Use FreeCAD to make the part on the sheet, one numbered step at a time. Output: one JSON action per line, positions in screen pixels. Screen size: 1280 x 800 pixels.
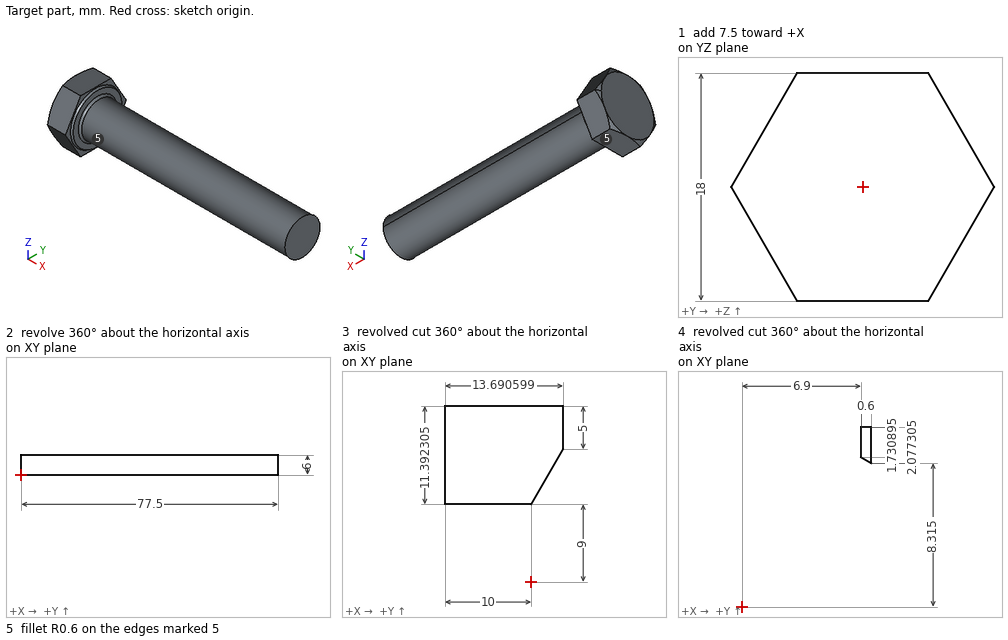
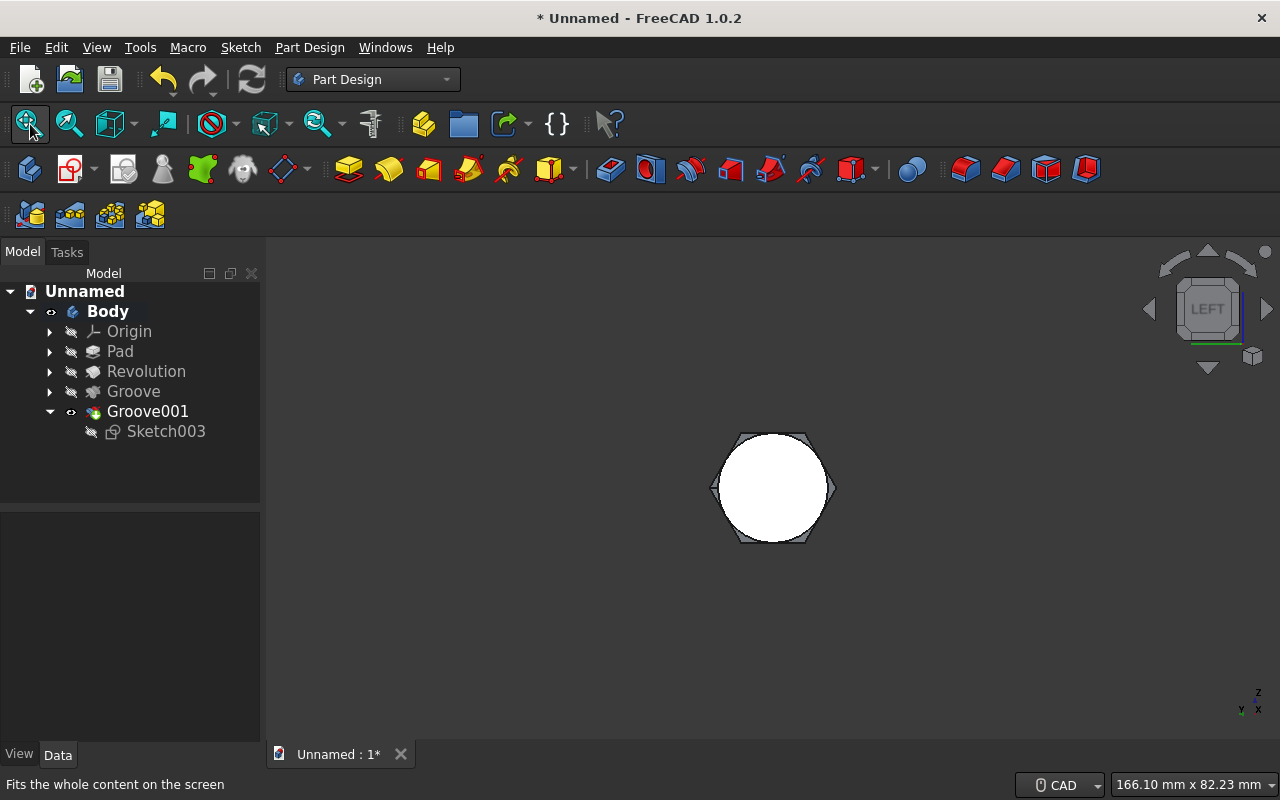
{"action": "left_click", "coordinate": [30, 124]}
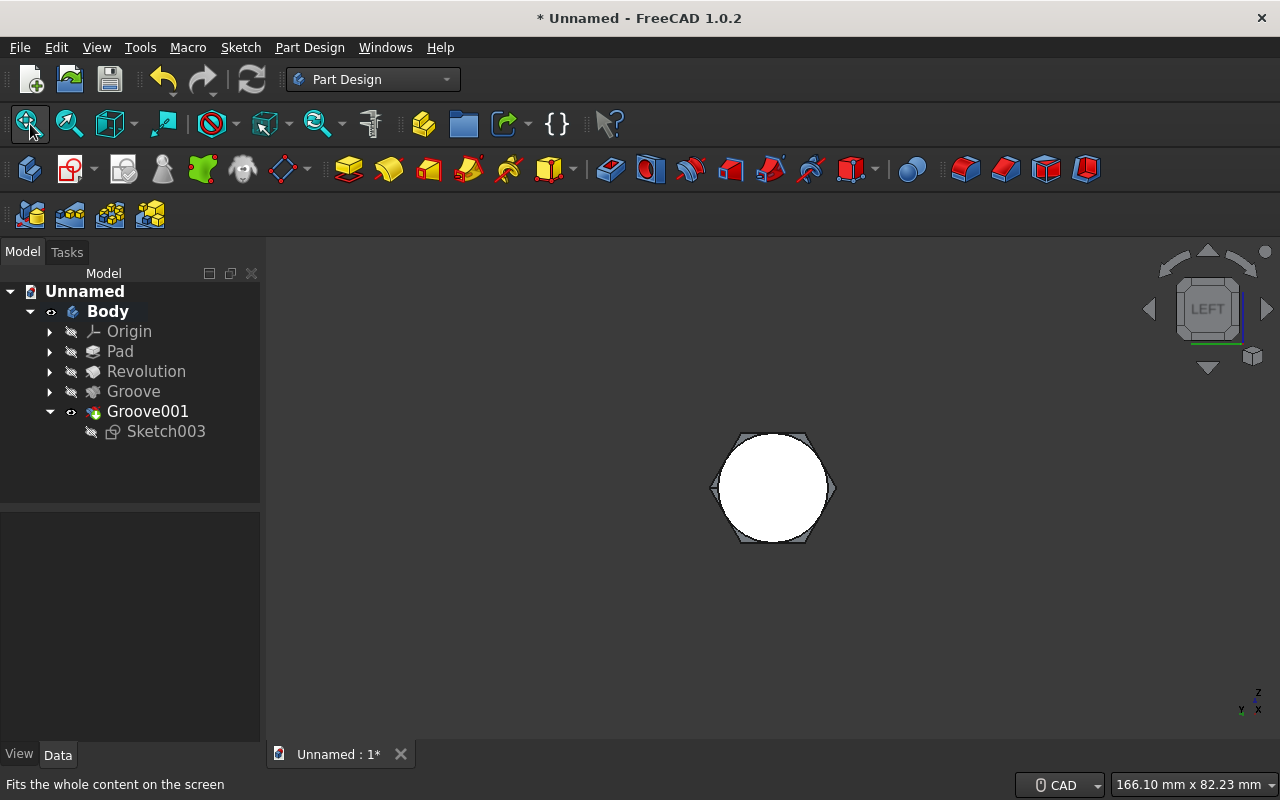
{"action": "key", "text": "v 3"}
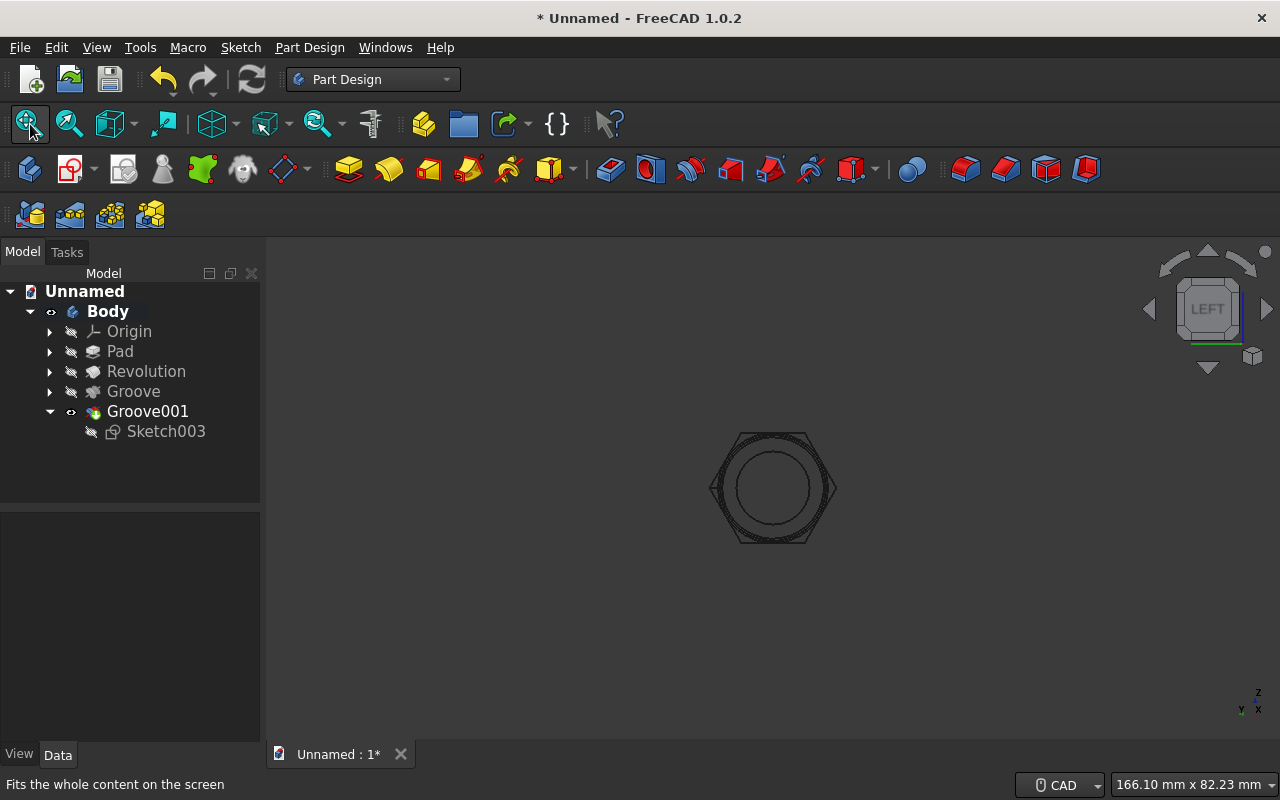
{"action": "key", "text": "0"}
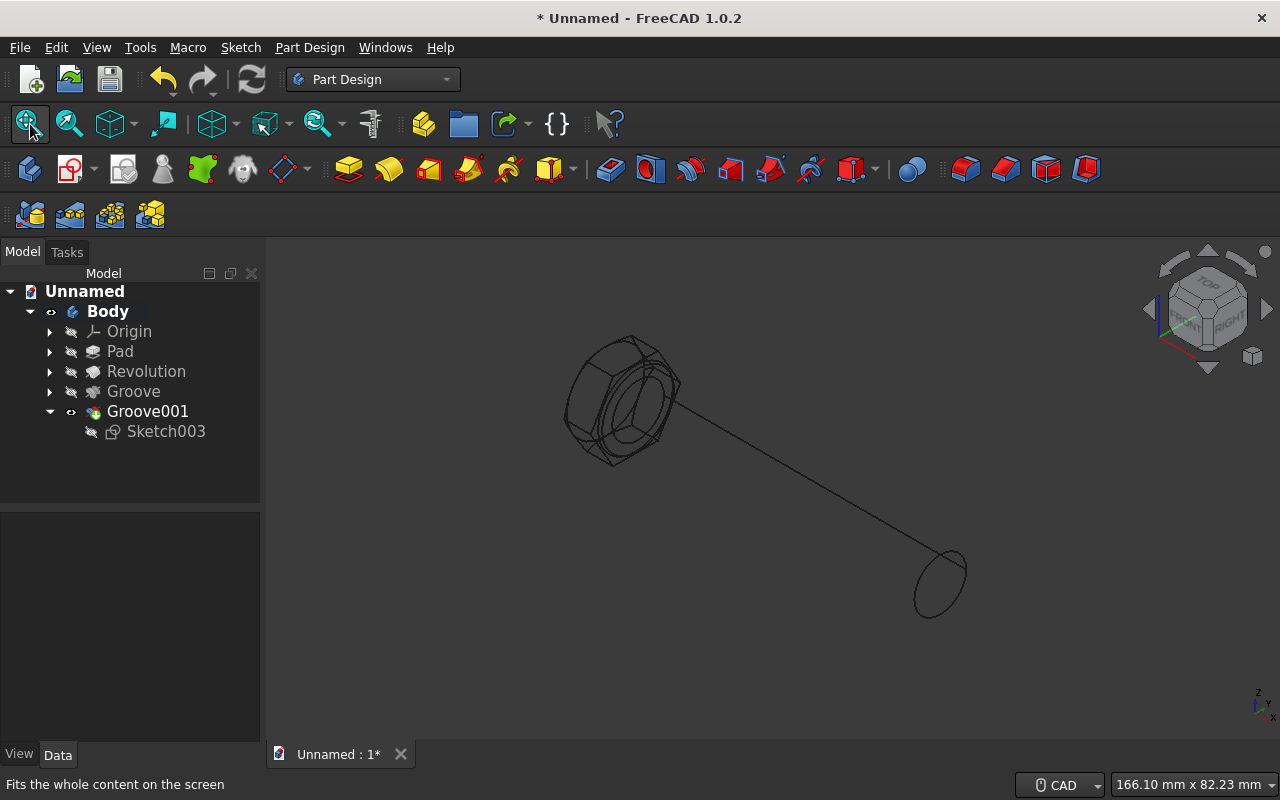
{"action": "left_click", "coordinate": [612, 424]}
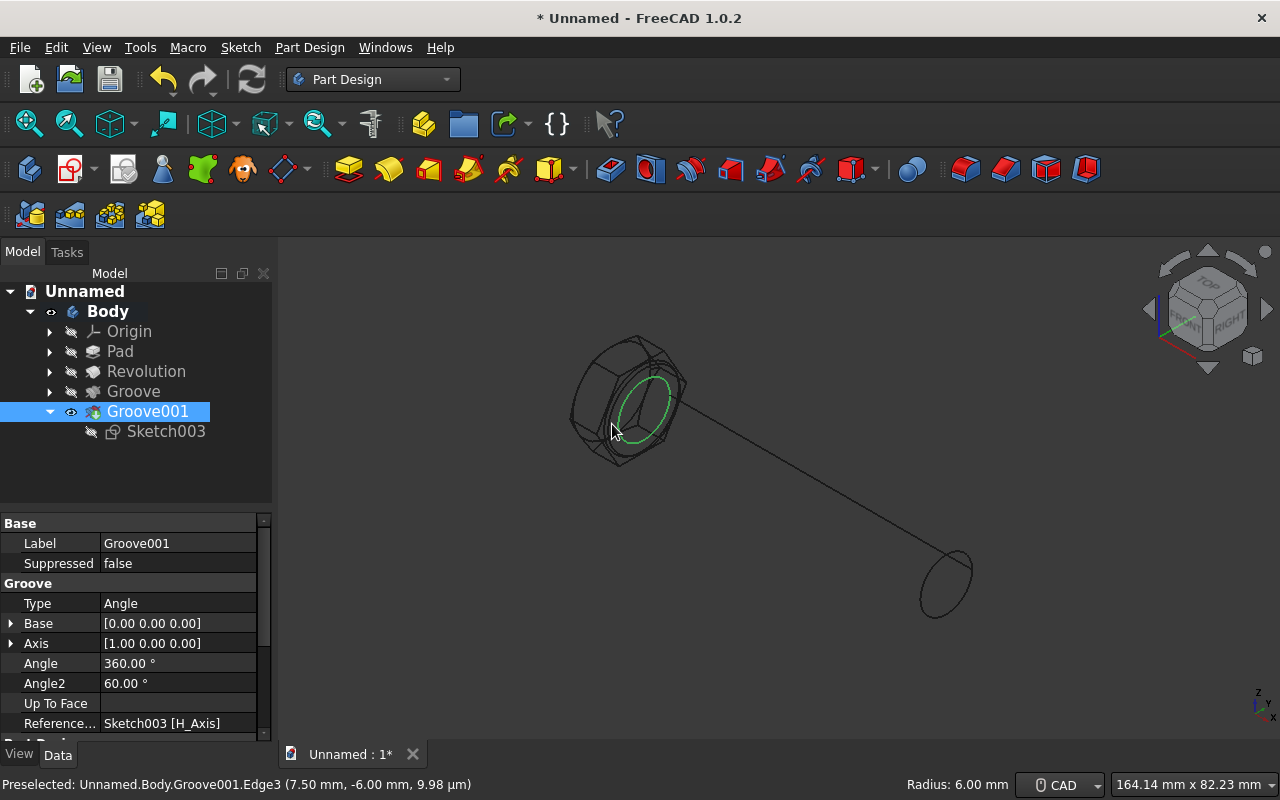
{"action": "key", "text": "v 1"}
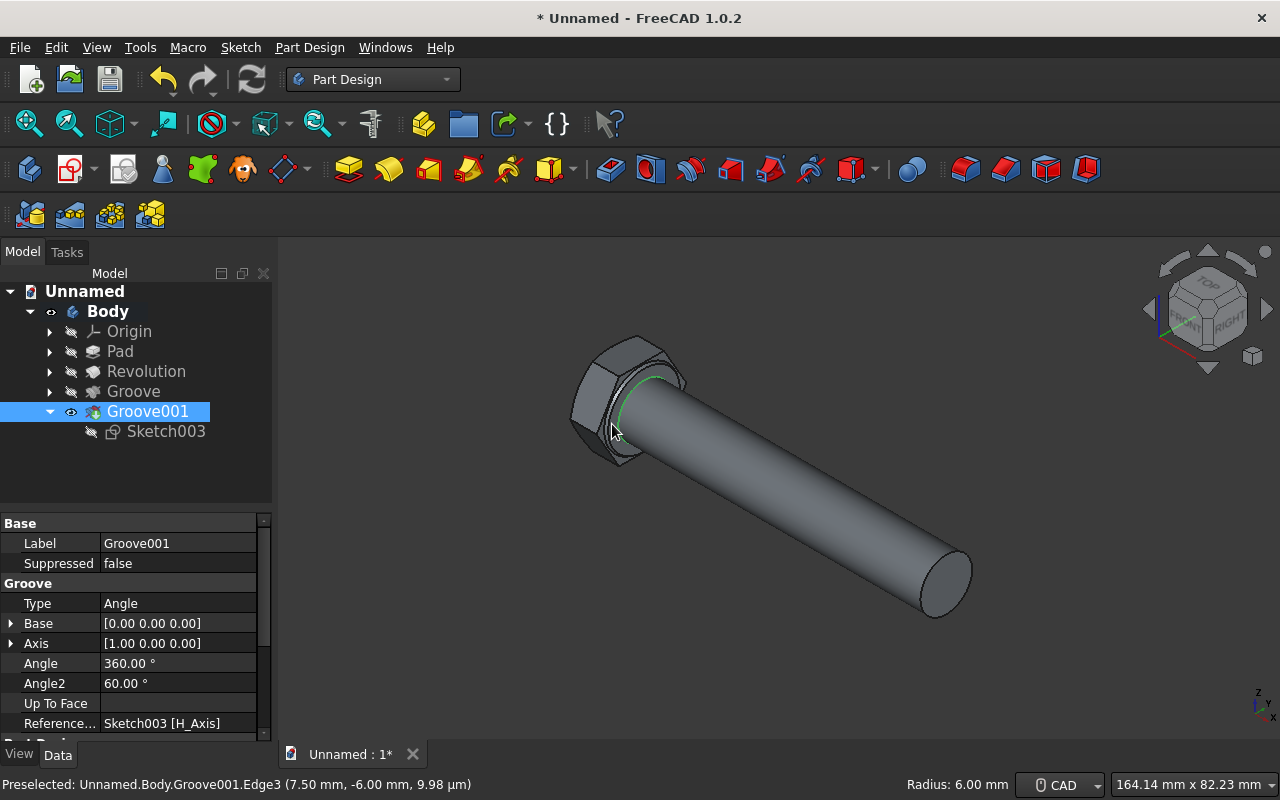
{"action": "left_click", "coordinate": [966, 170]}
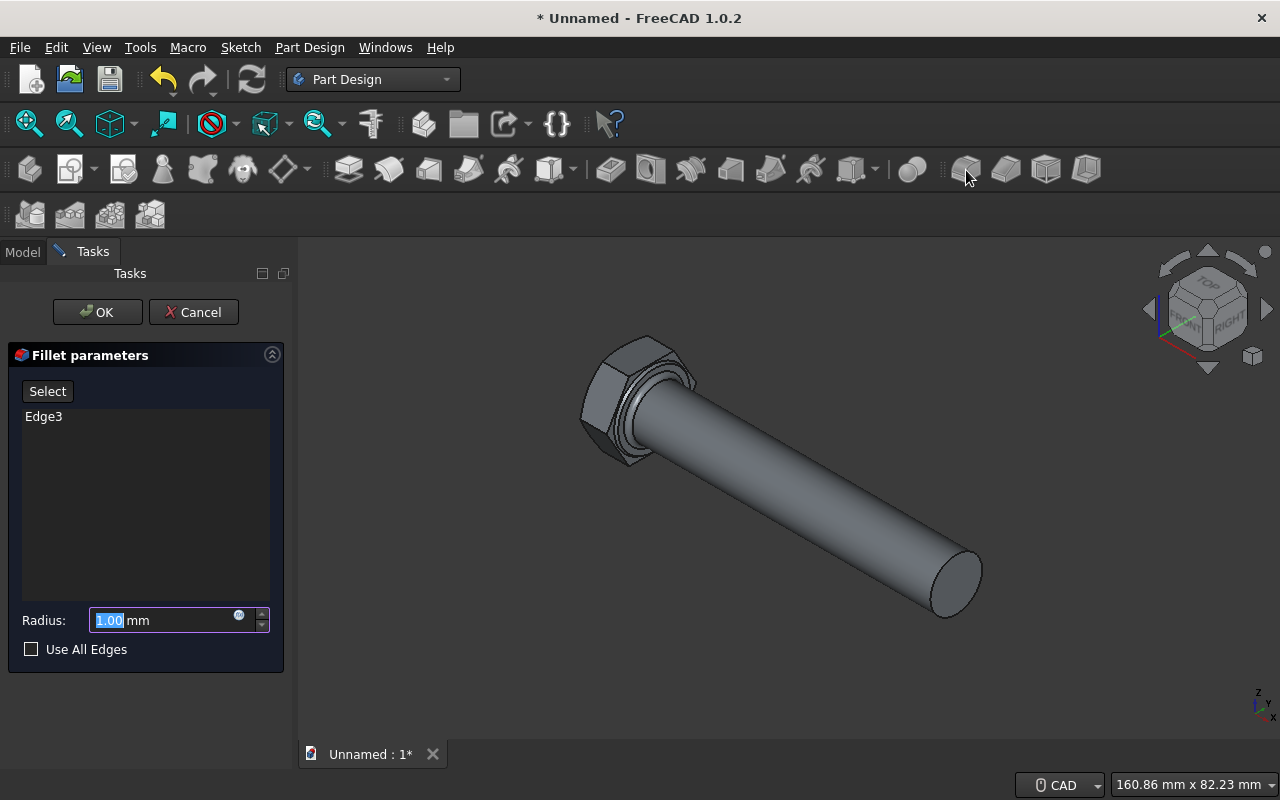
{"action": "type", "text": "0.6"}
{"action": "key", "text": "Tab"}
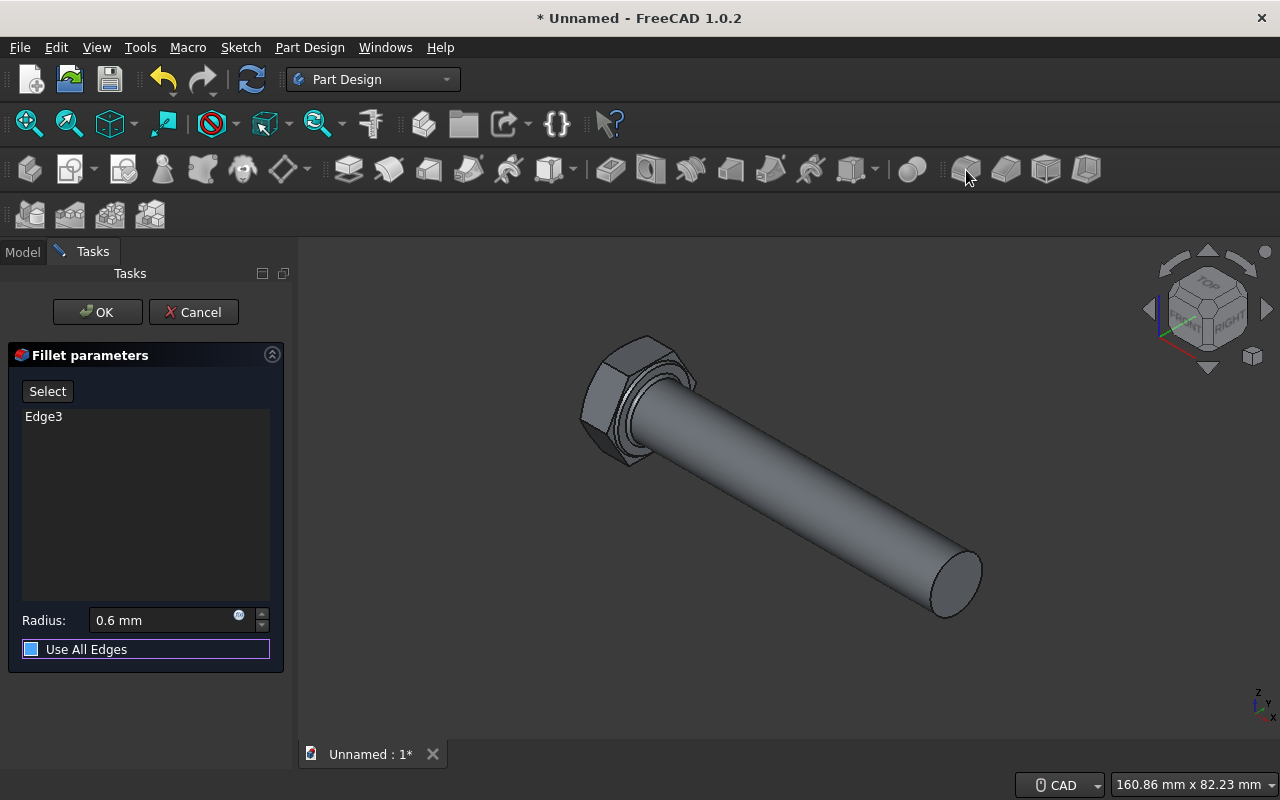
{"action": "left_click", "coordinate": [98, 312]}